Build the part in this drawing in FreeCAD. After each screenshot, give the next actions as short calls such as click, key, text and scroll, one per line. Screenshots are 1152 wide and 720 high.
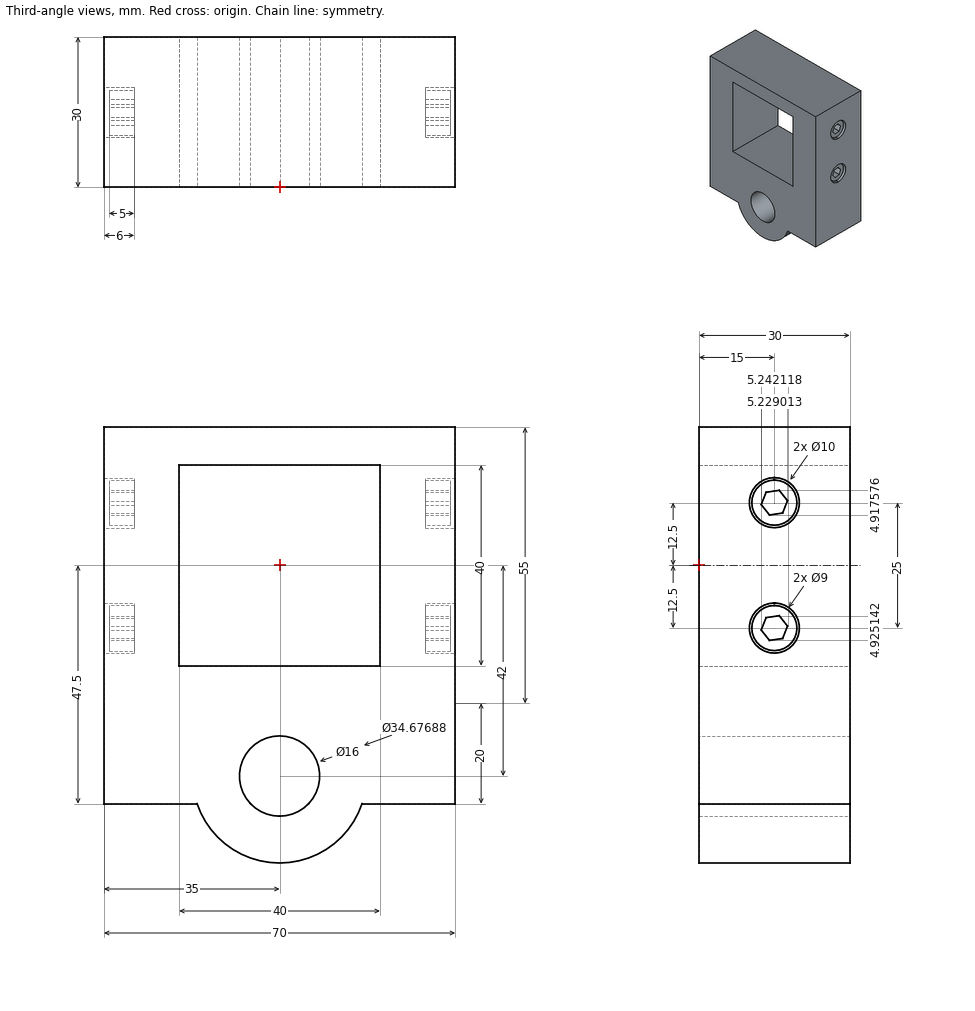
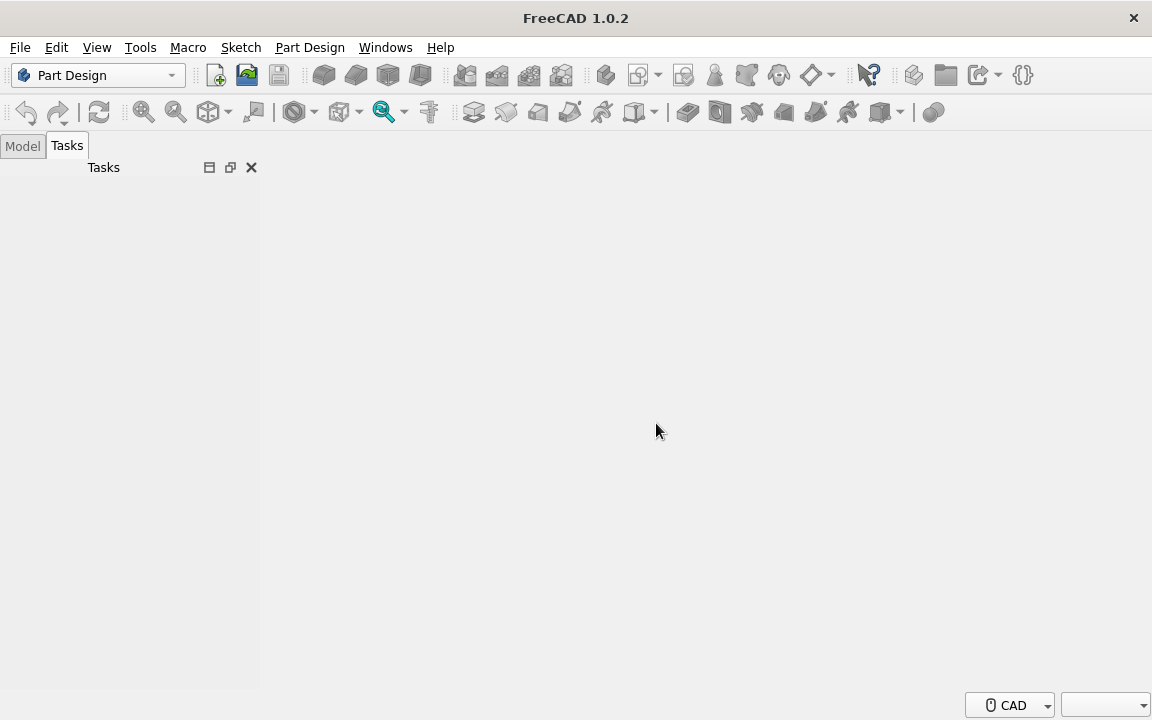
click(216, 76)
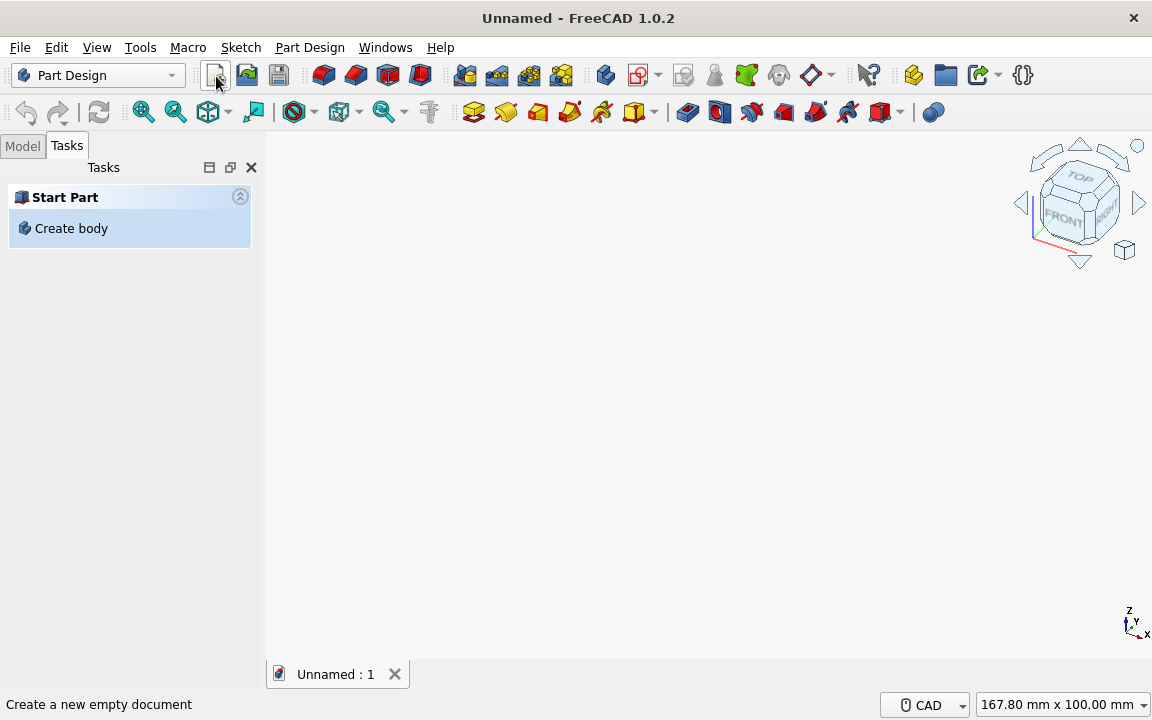
click(638, 76)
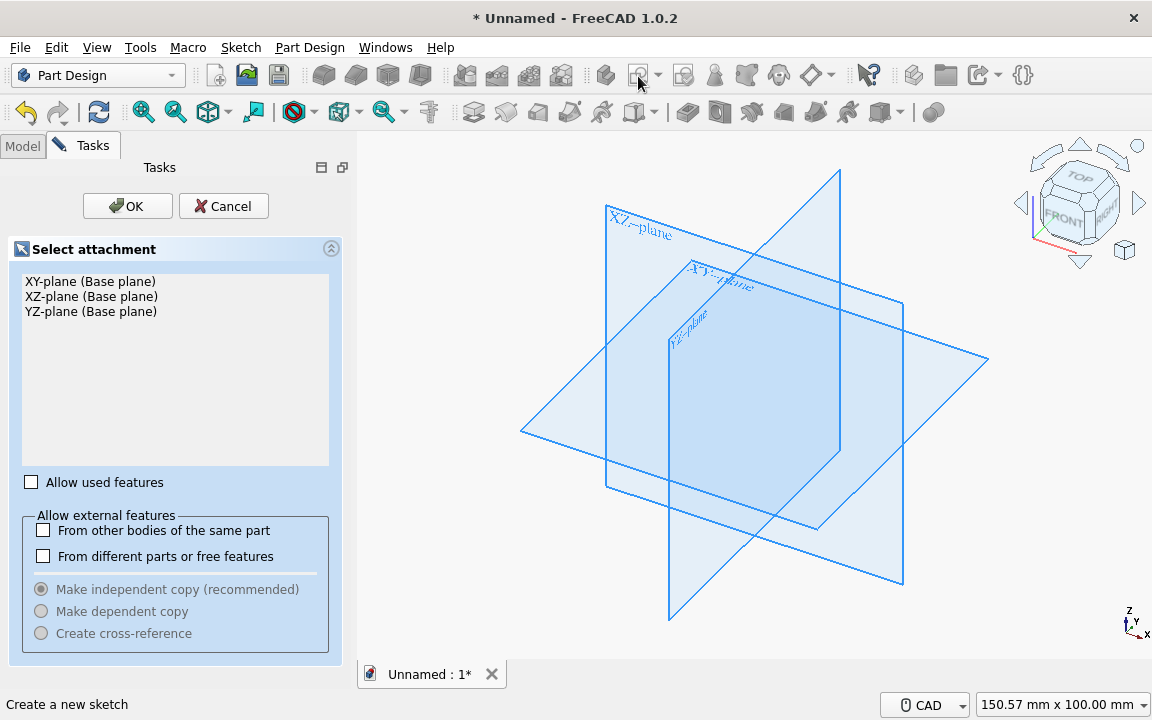
click(82, 296)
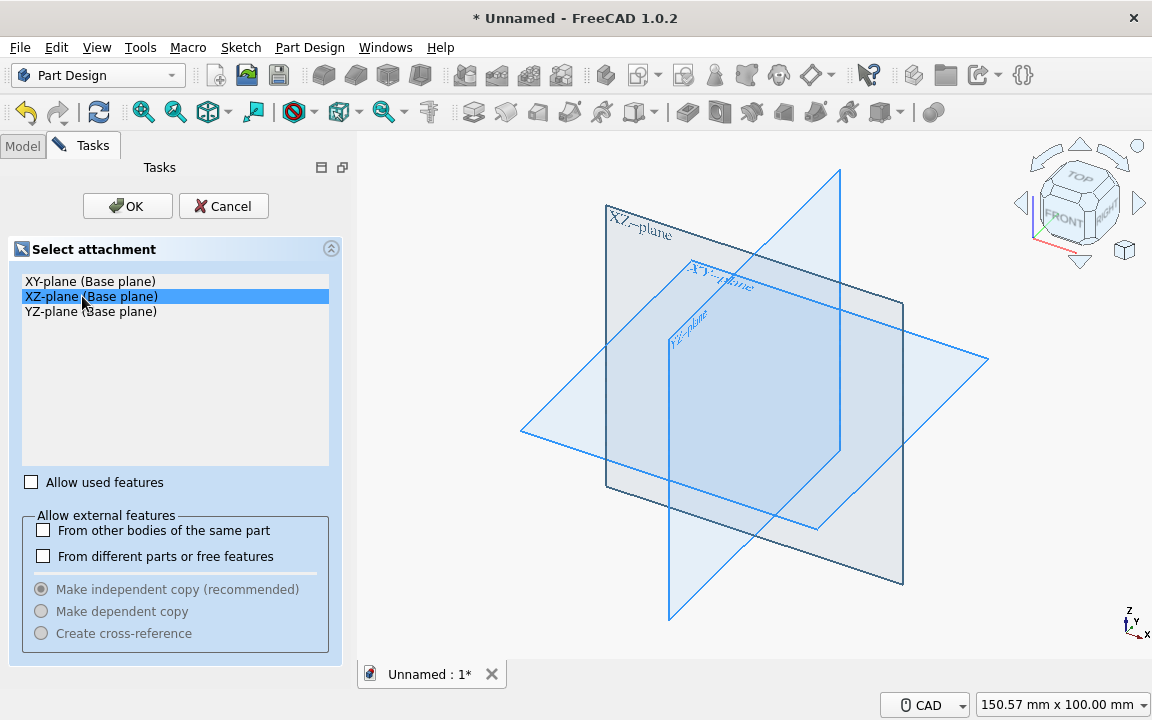
click(128, 206)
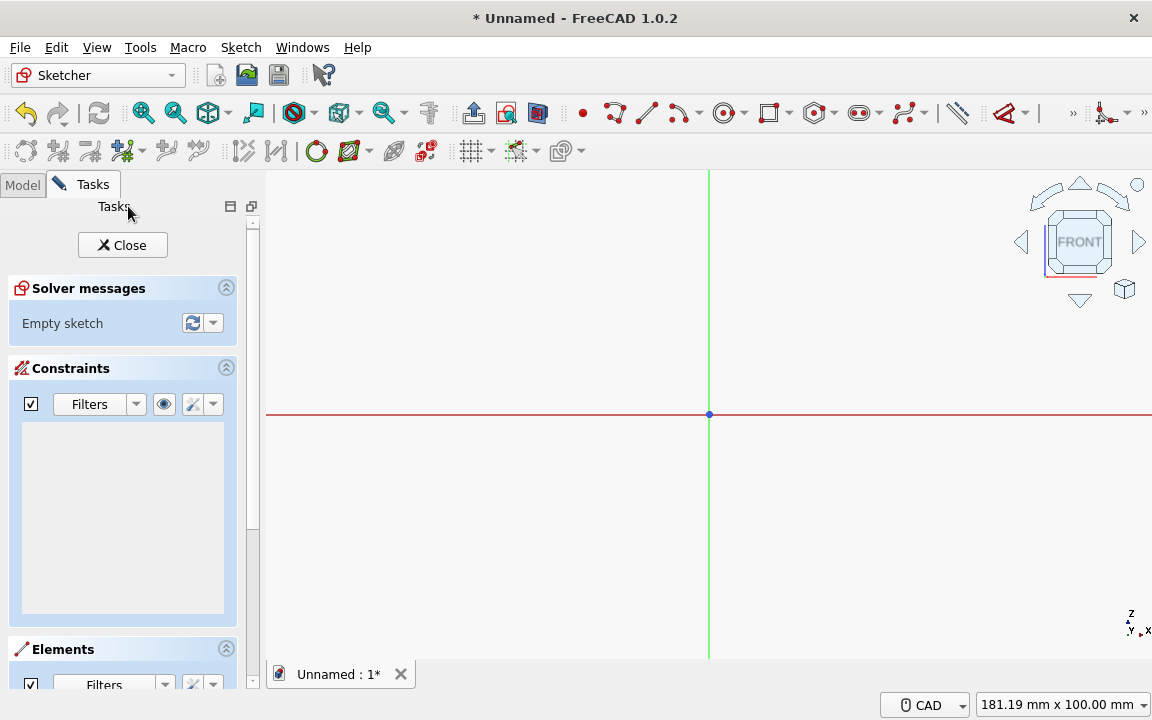
key(g)
key(v)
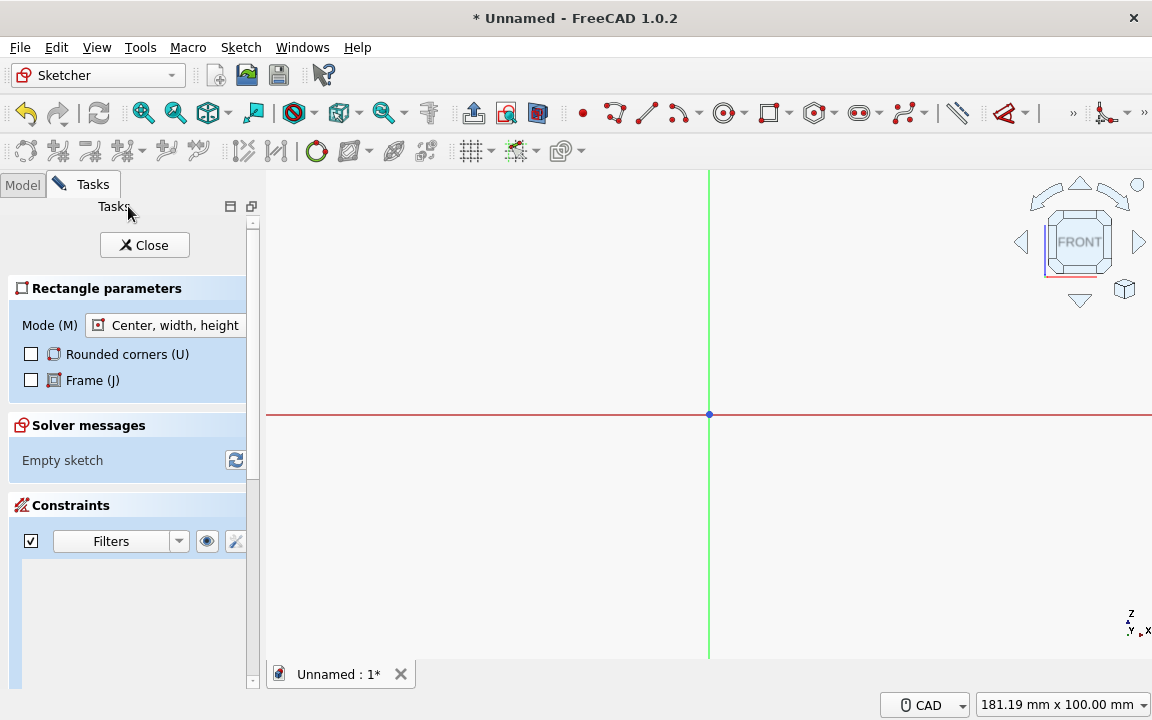
click(709, 414)
move(880, 280)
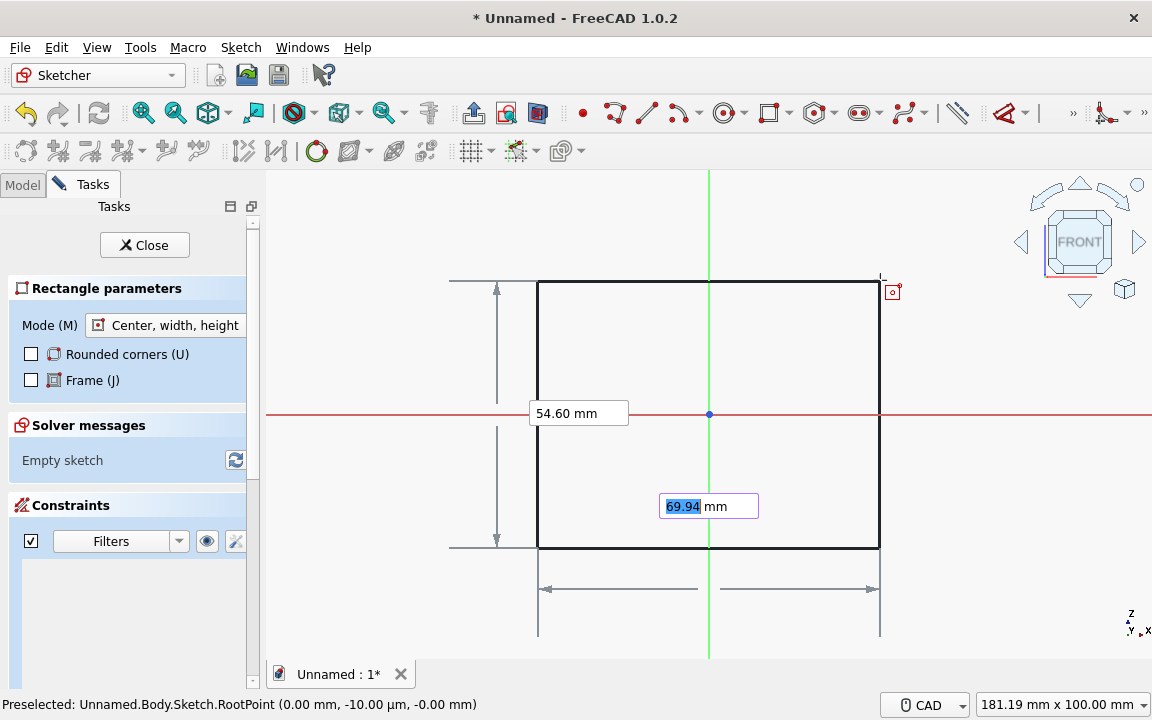
text(70)
key(Tab)
text(55)
key(Return)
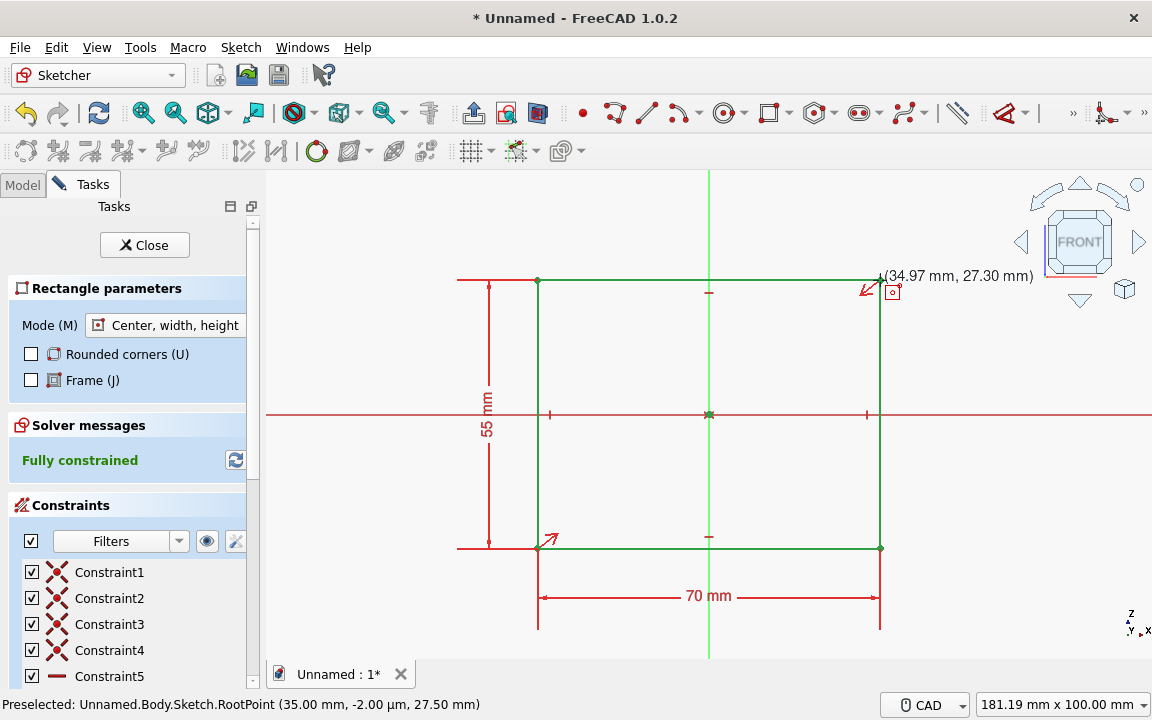
click(709, 414)
move(807, 317)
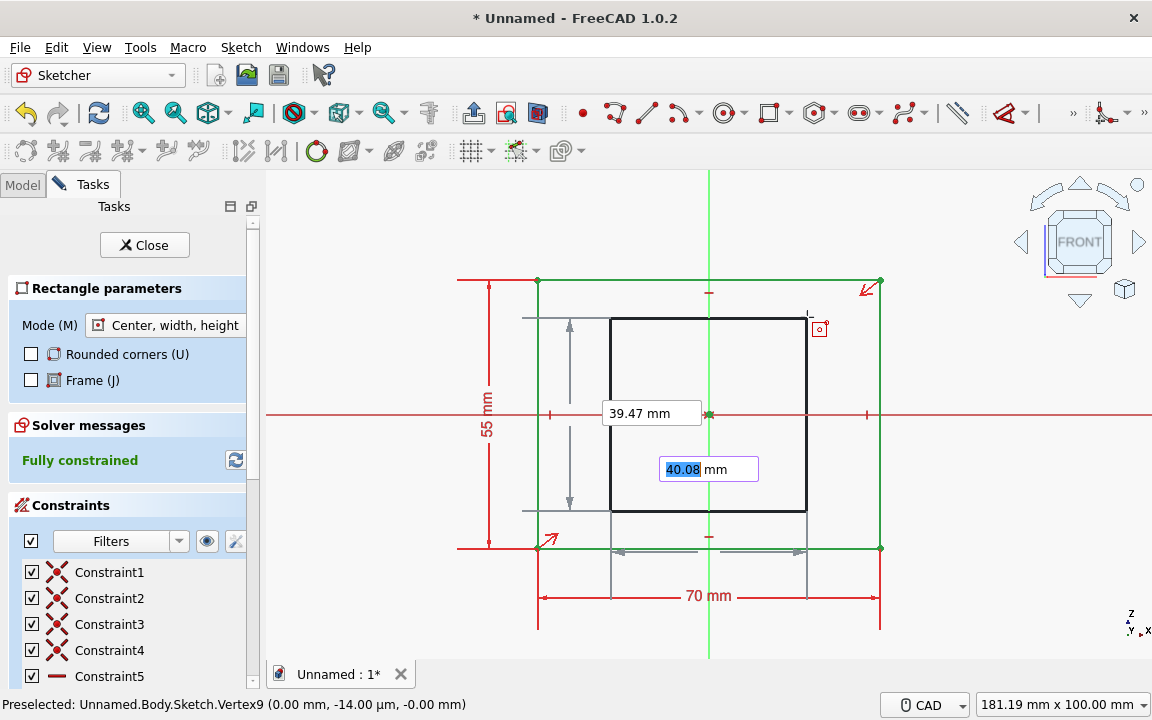
text(40)
key(Tab)
text(40)
key(Return)
key(Escape)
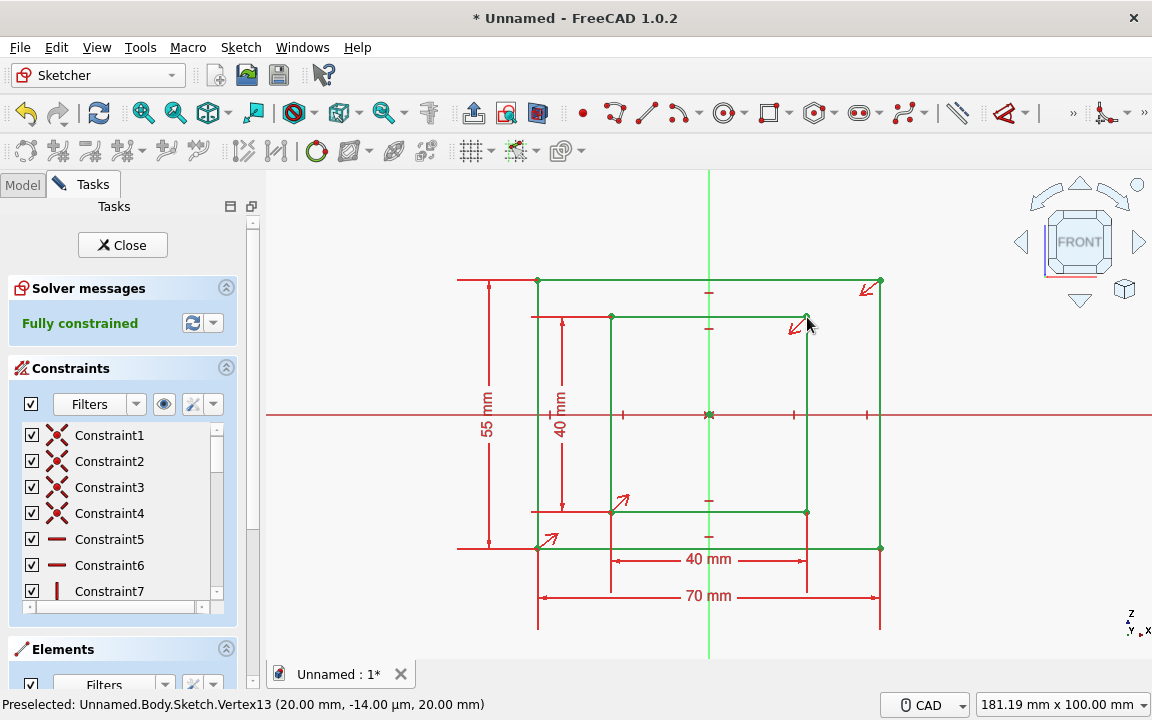
click(123, 245)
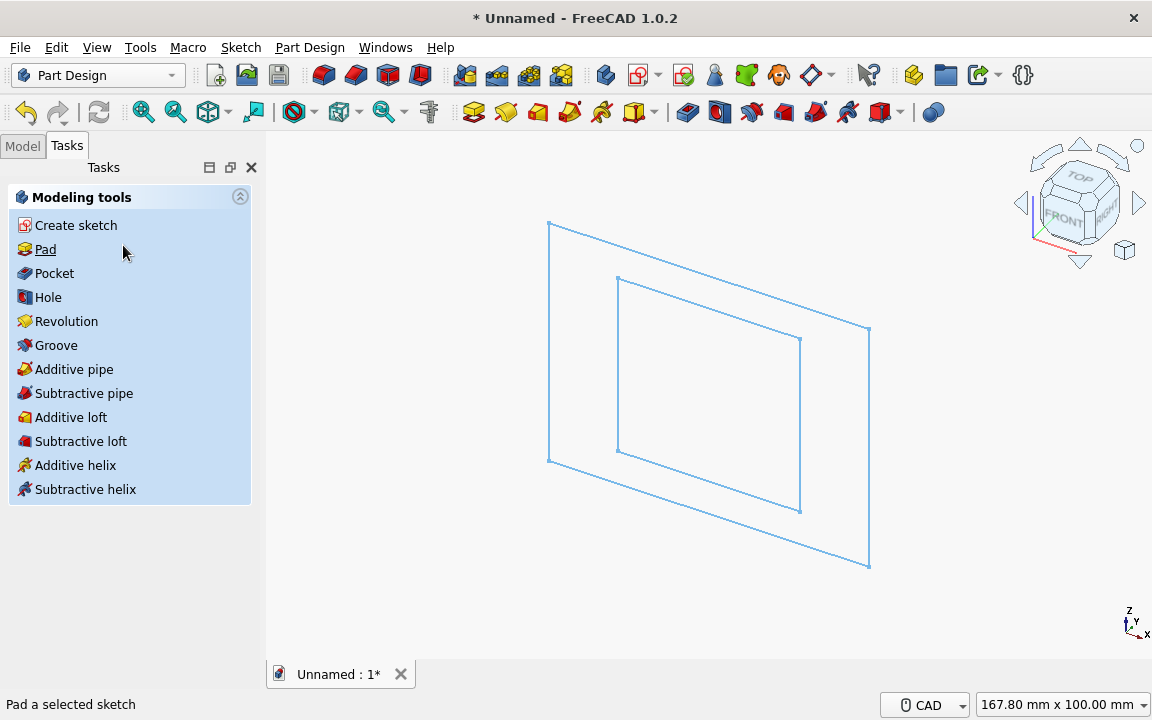
click(474, 112)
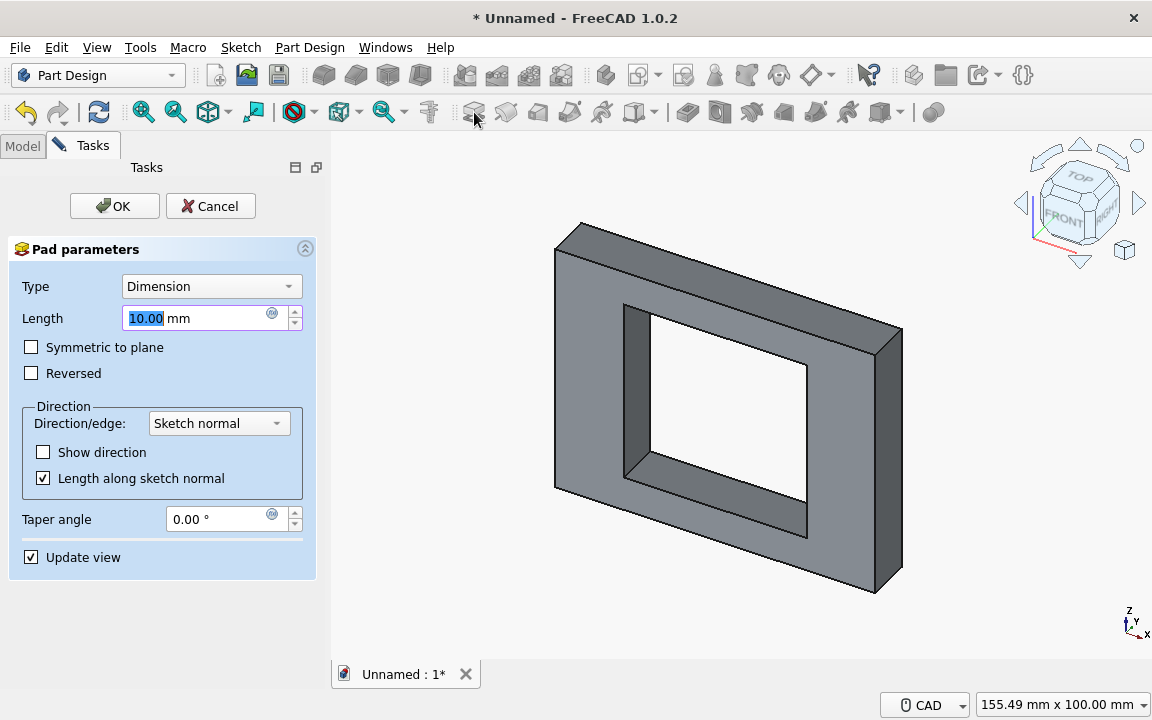
text(30)
key(Tab)